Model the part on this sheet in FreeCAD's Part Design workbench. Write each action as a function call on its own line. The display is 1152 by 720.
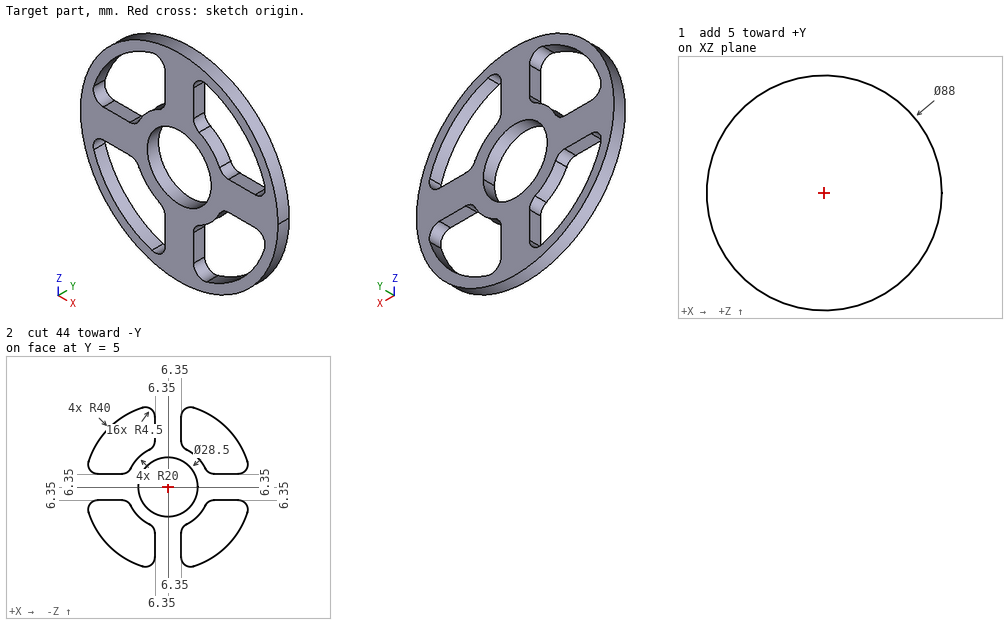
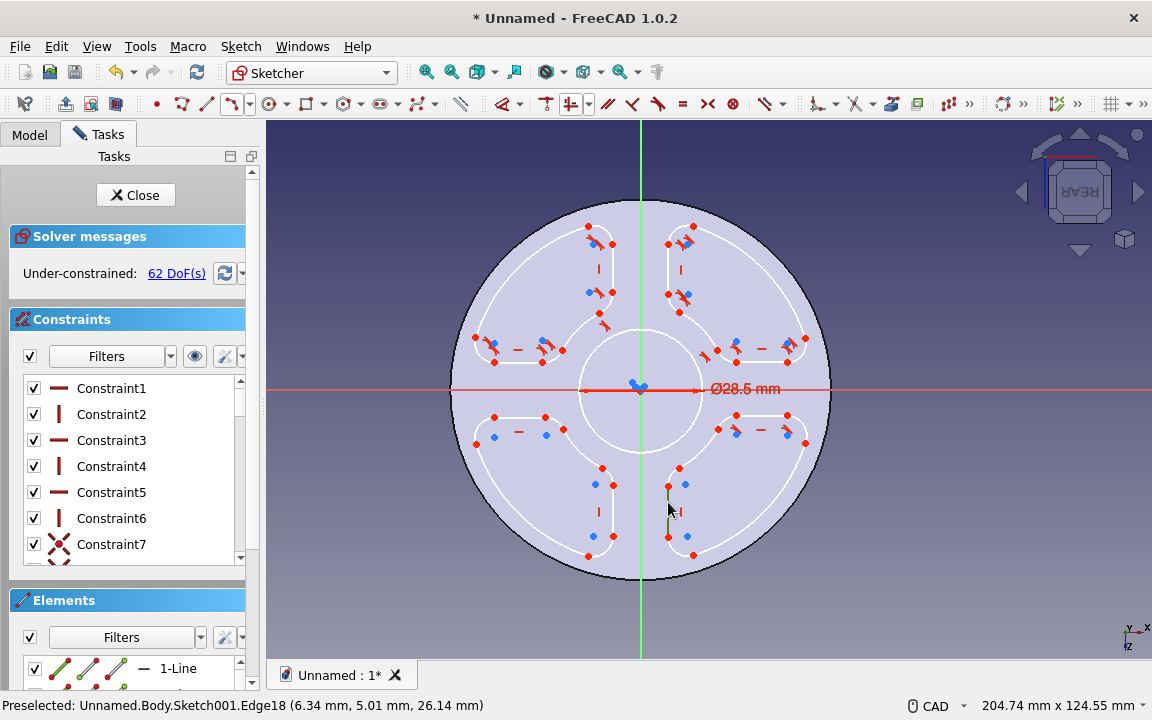
scroll(671, 475, up, 2)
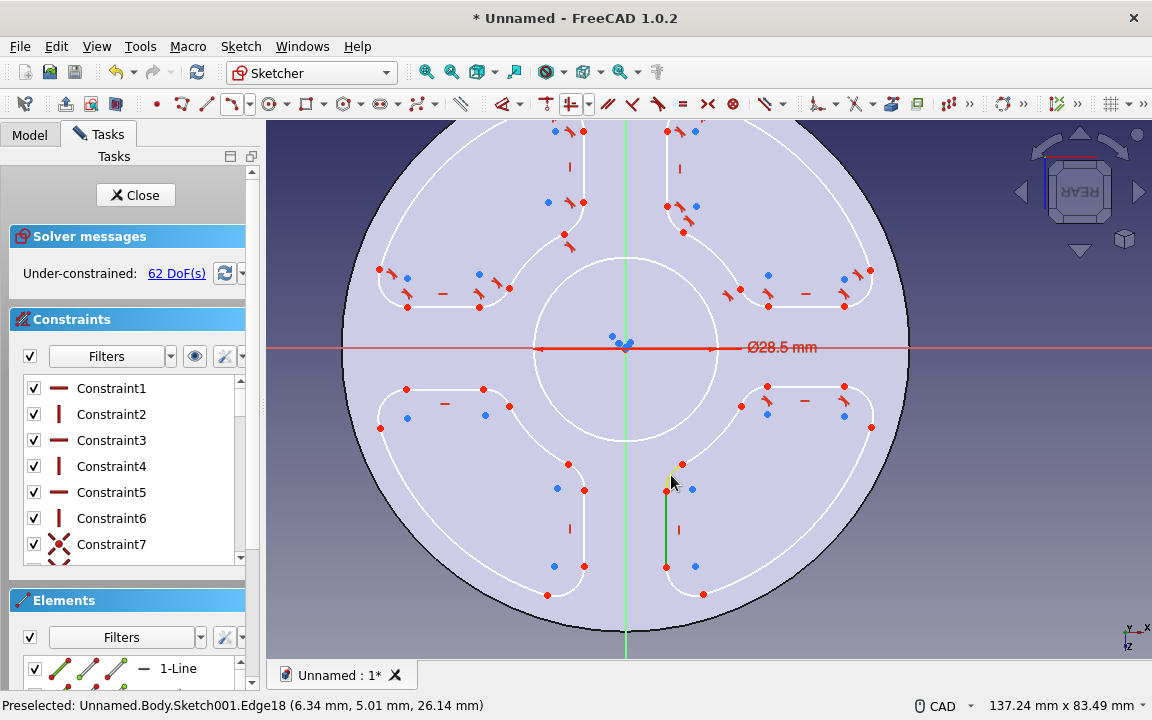
click(670, 475)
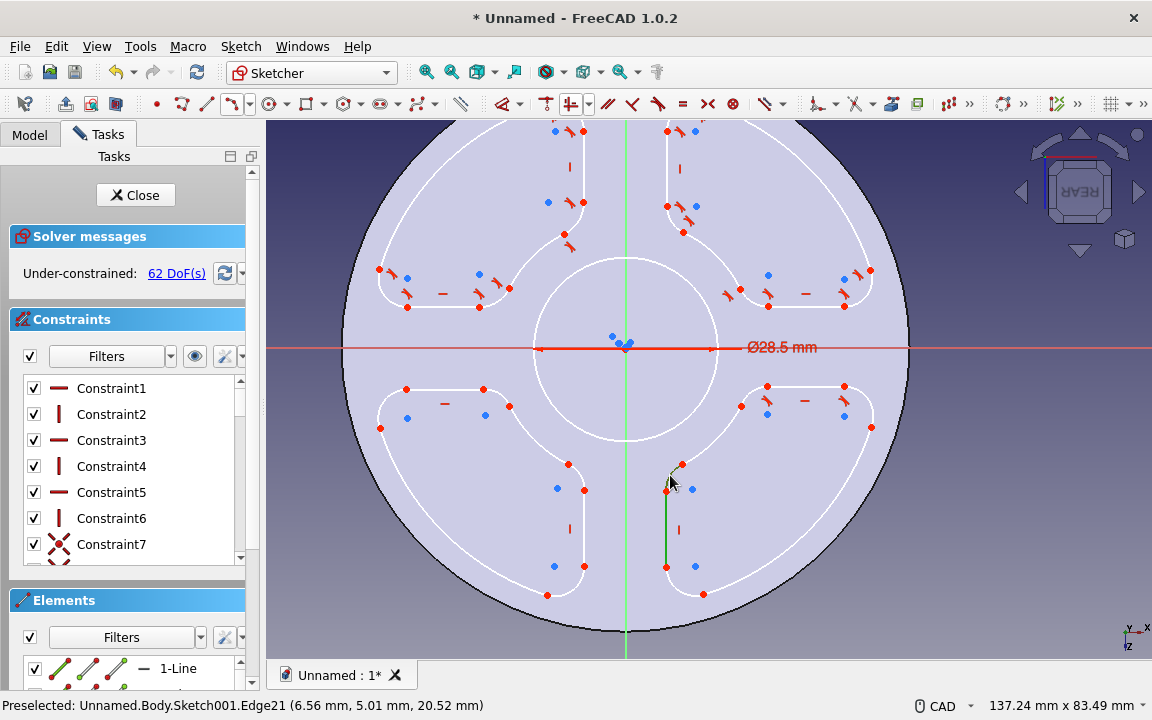
key(t)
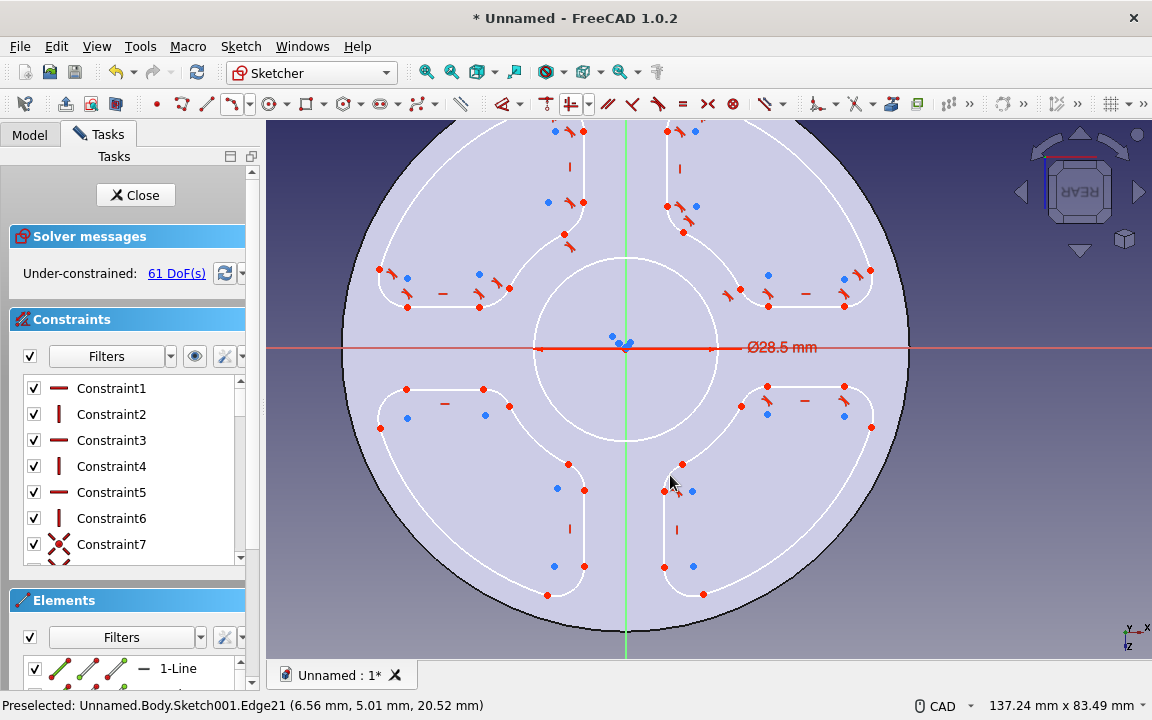
click(664, 514)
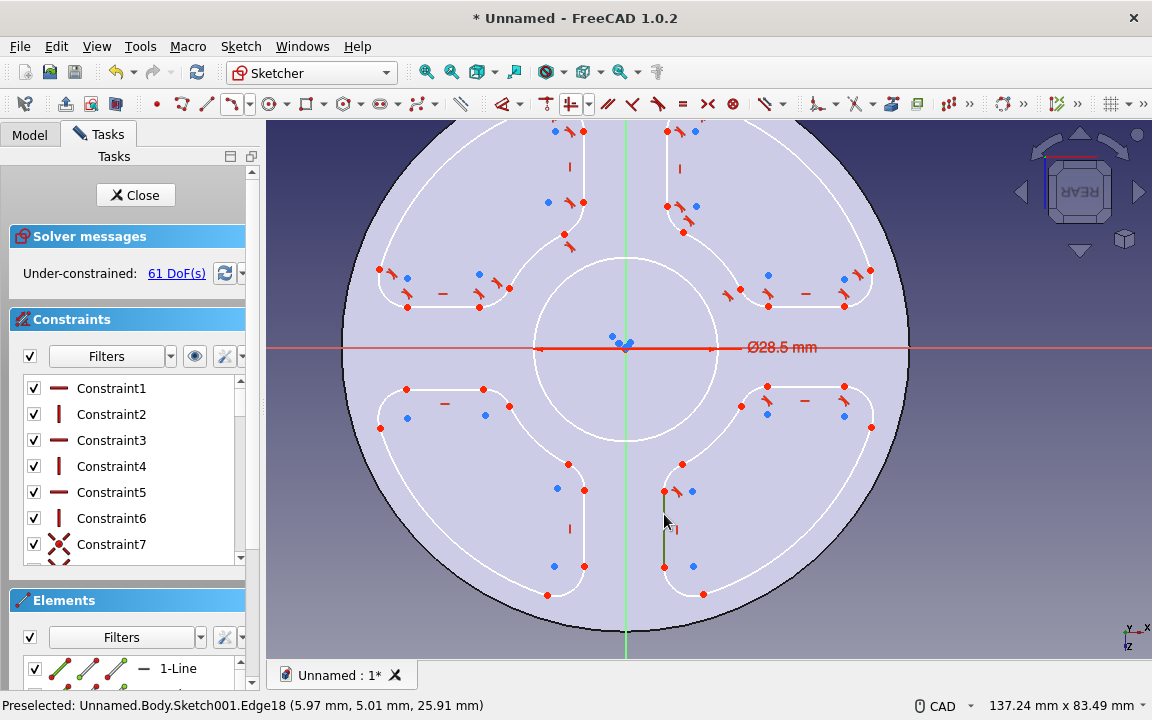
click(669, 583)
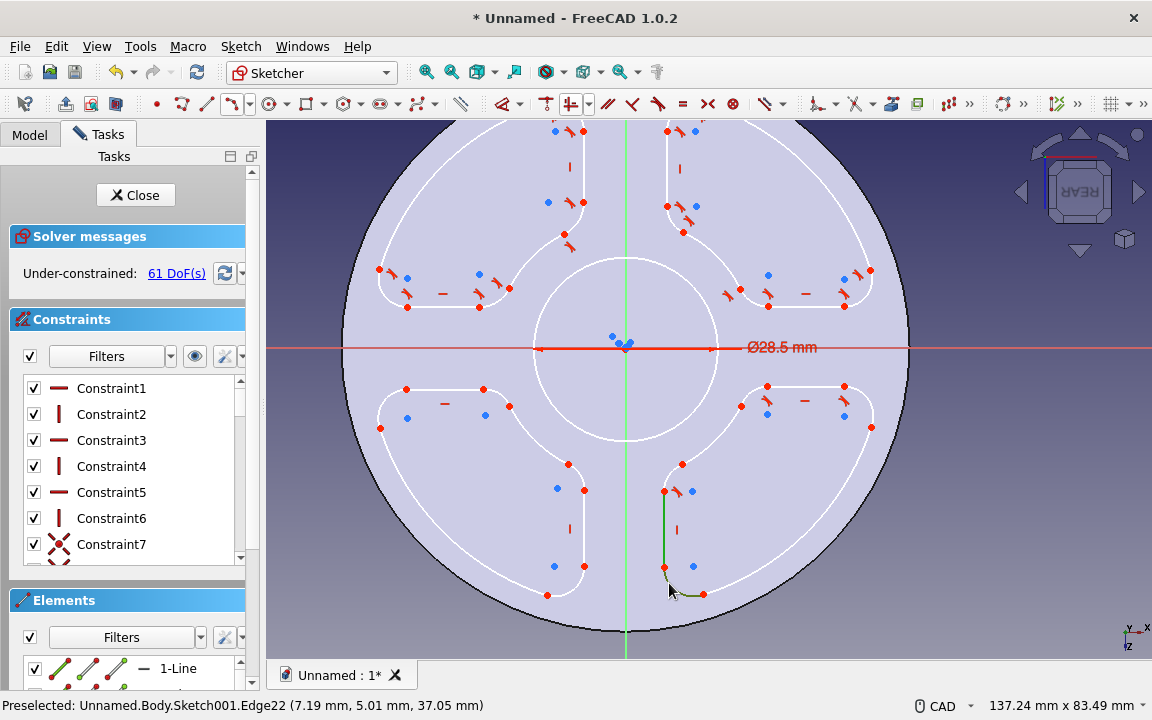
key(t)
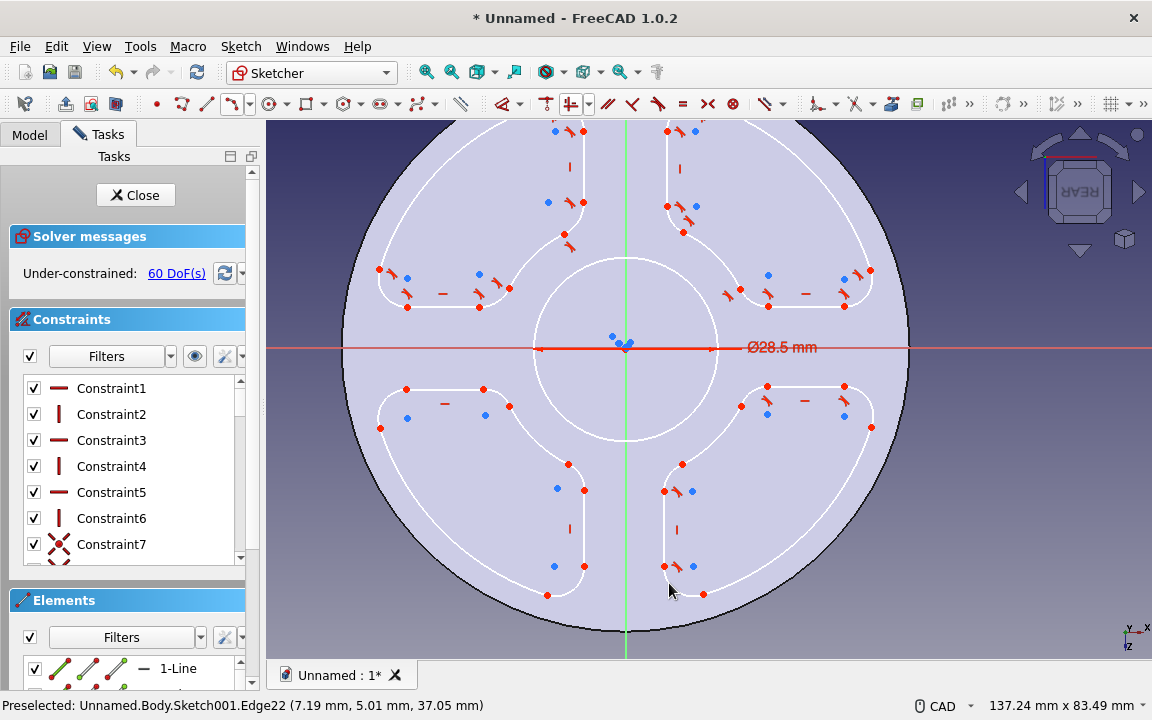
scroll(757, 389, up, 2)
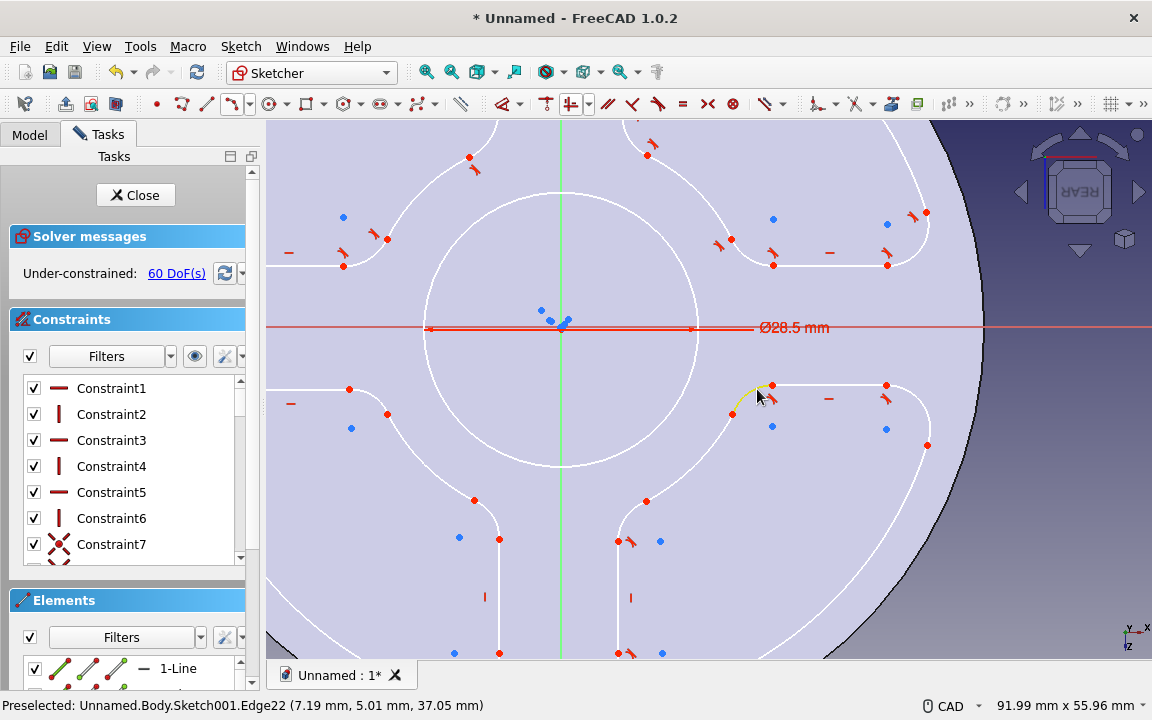
click(757, 388)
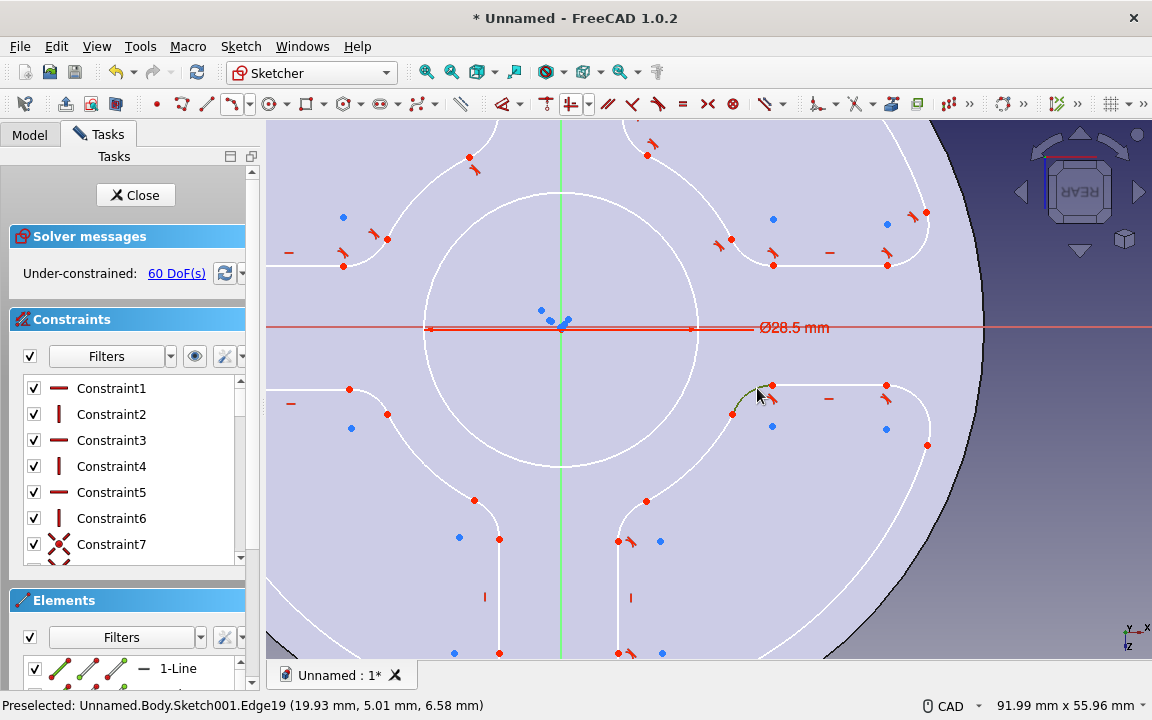
click(677, 481)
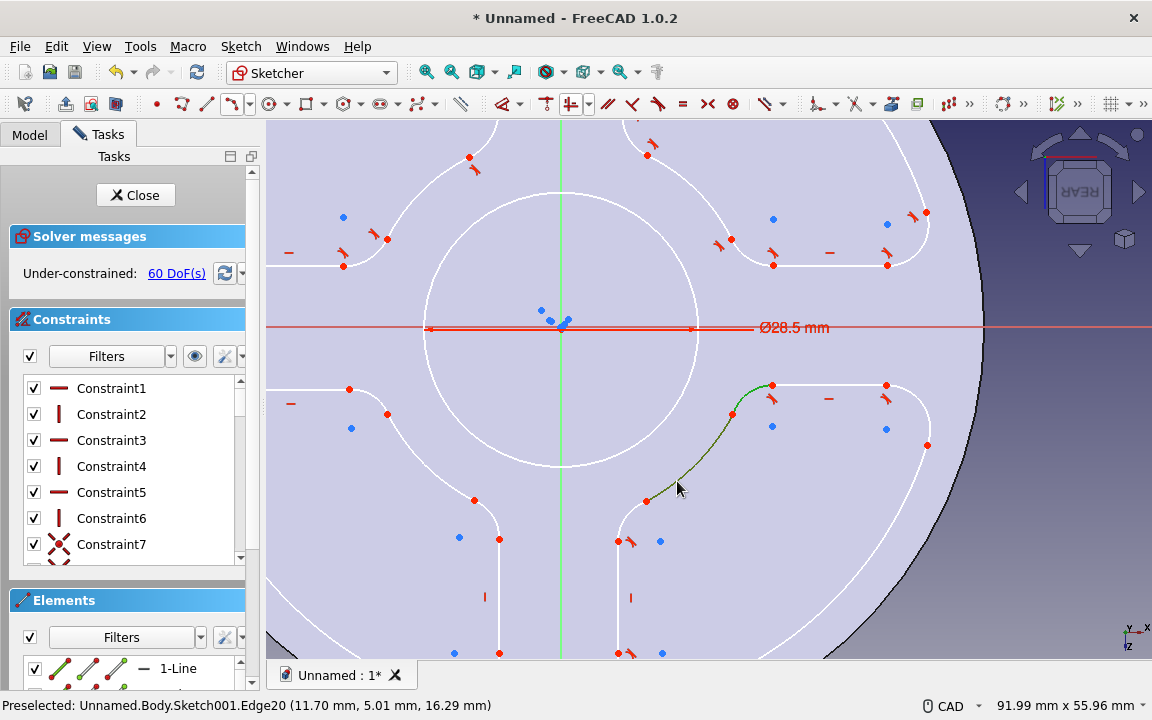
key(t)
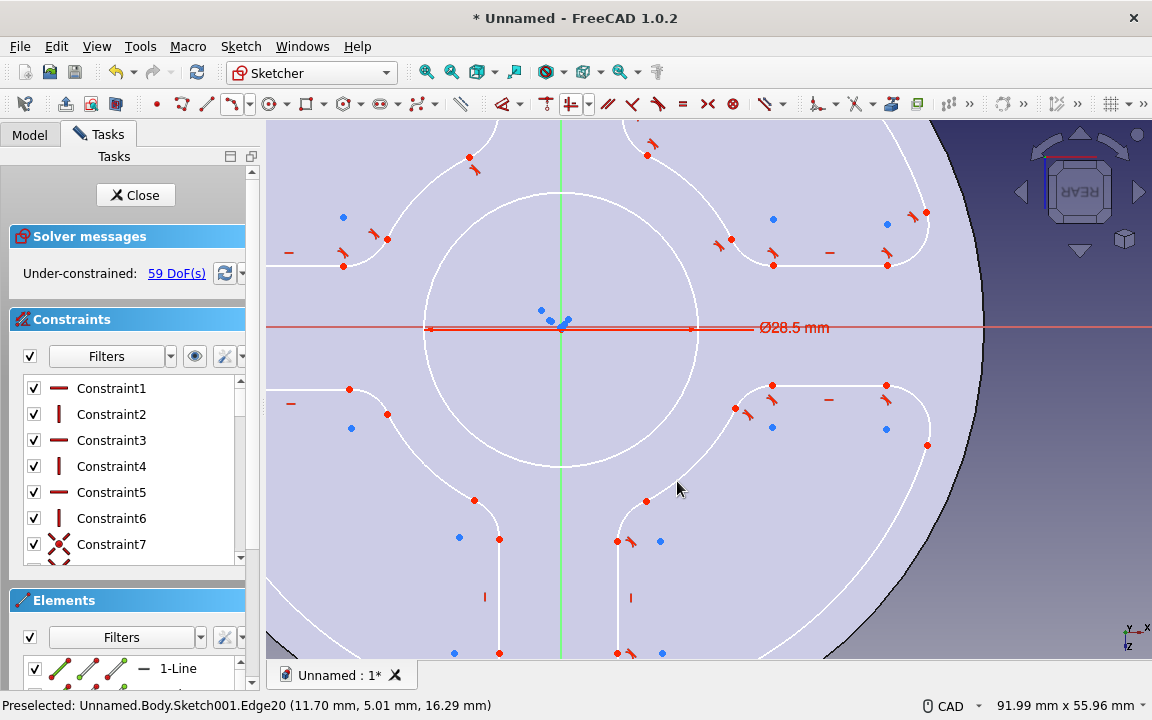
click(679, 479)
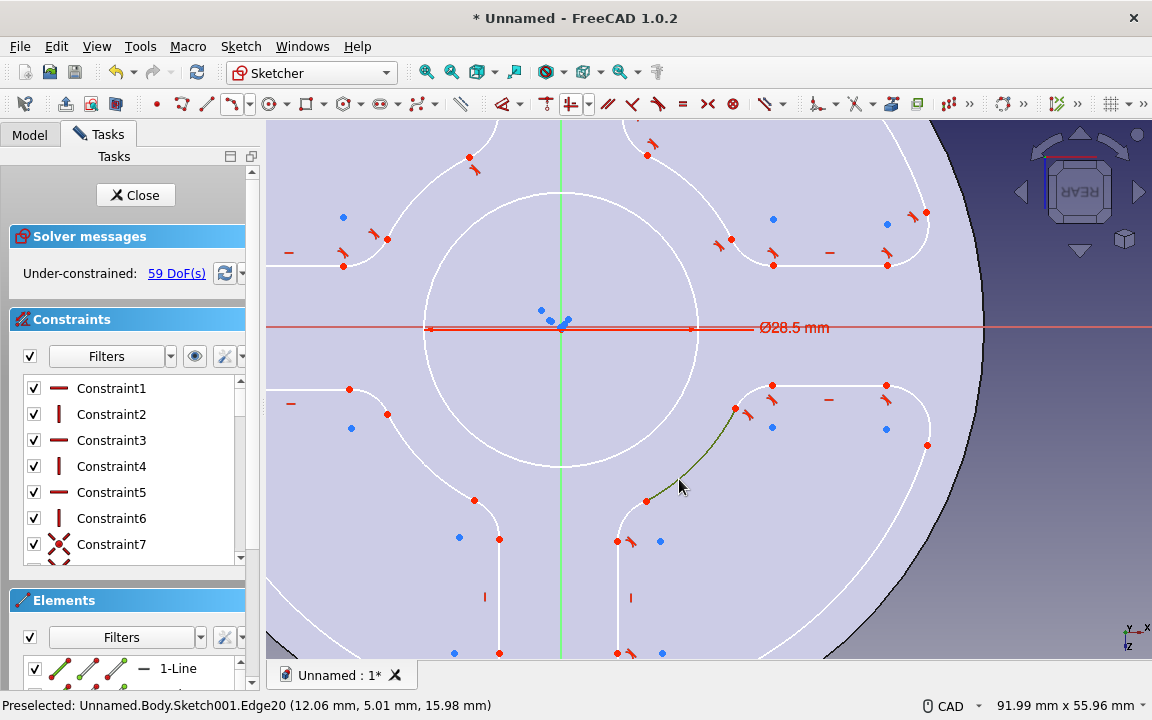
click(633, 509)